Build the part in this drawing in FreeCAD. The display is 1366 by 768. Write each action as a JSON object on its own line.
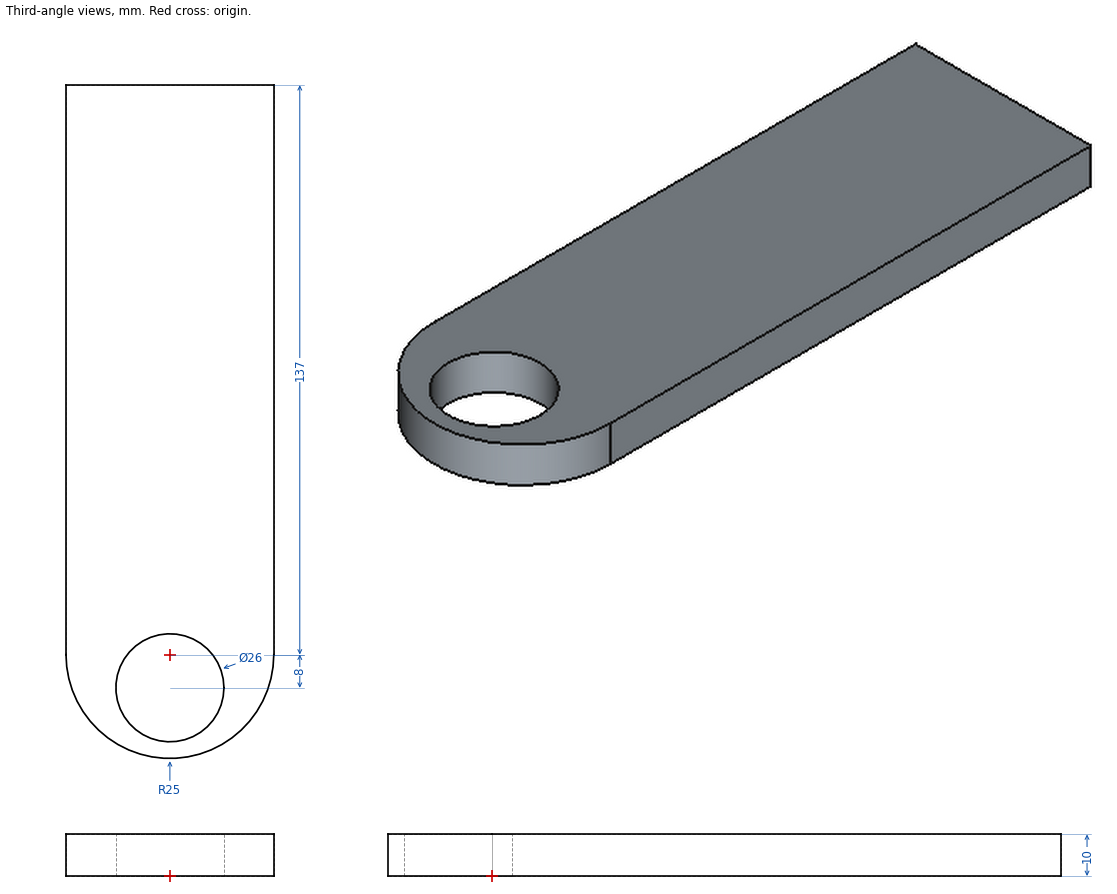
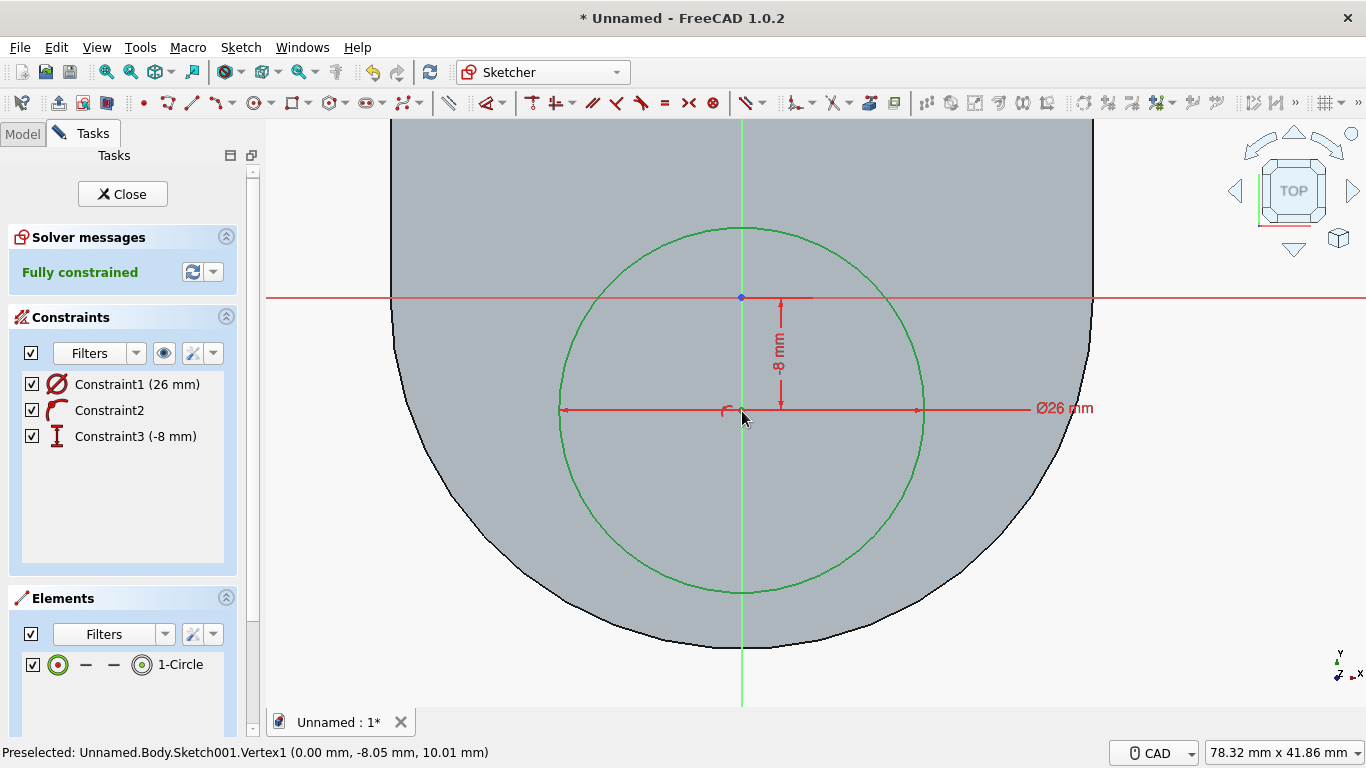
{"action": "left_click", "coordinate": [123, 194]}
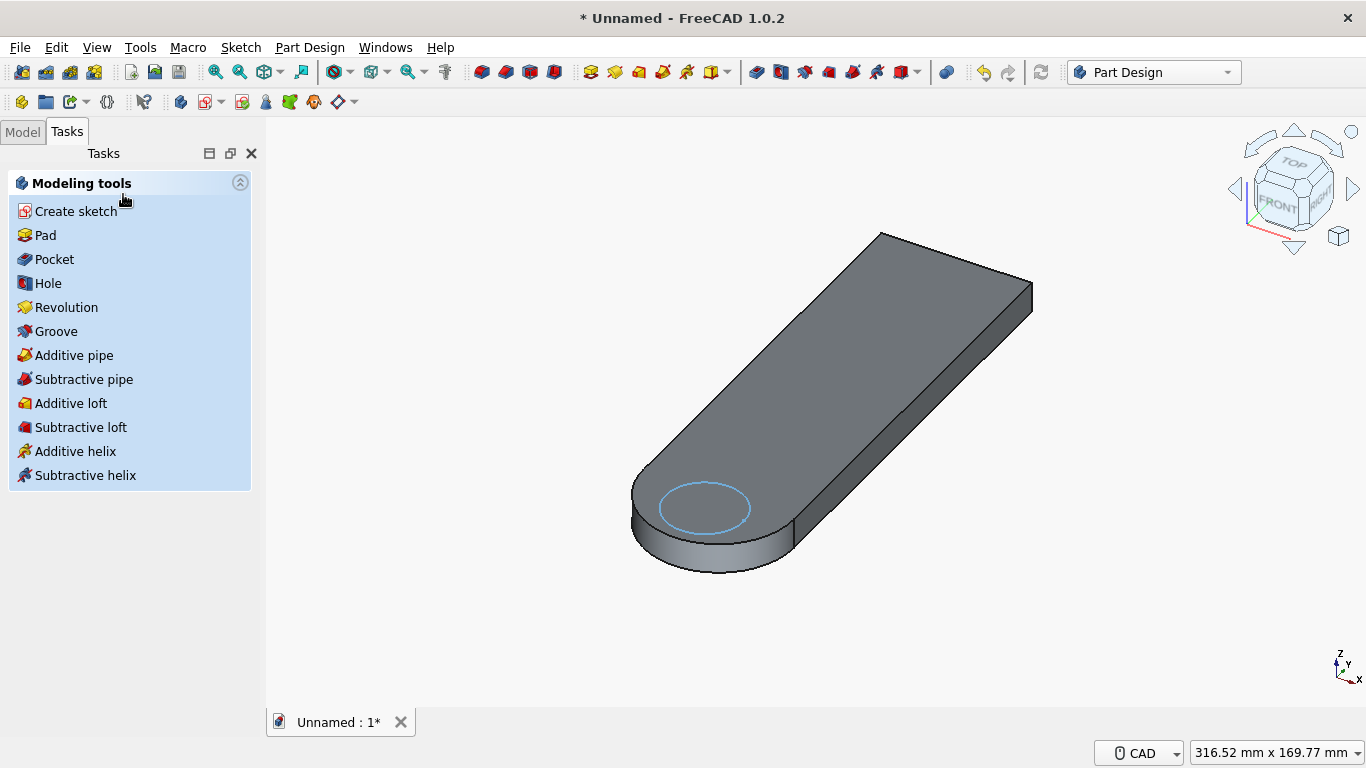
{"action": "left_click", "coordinate": [758, 72]}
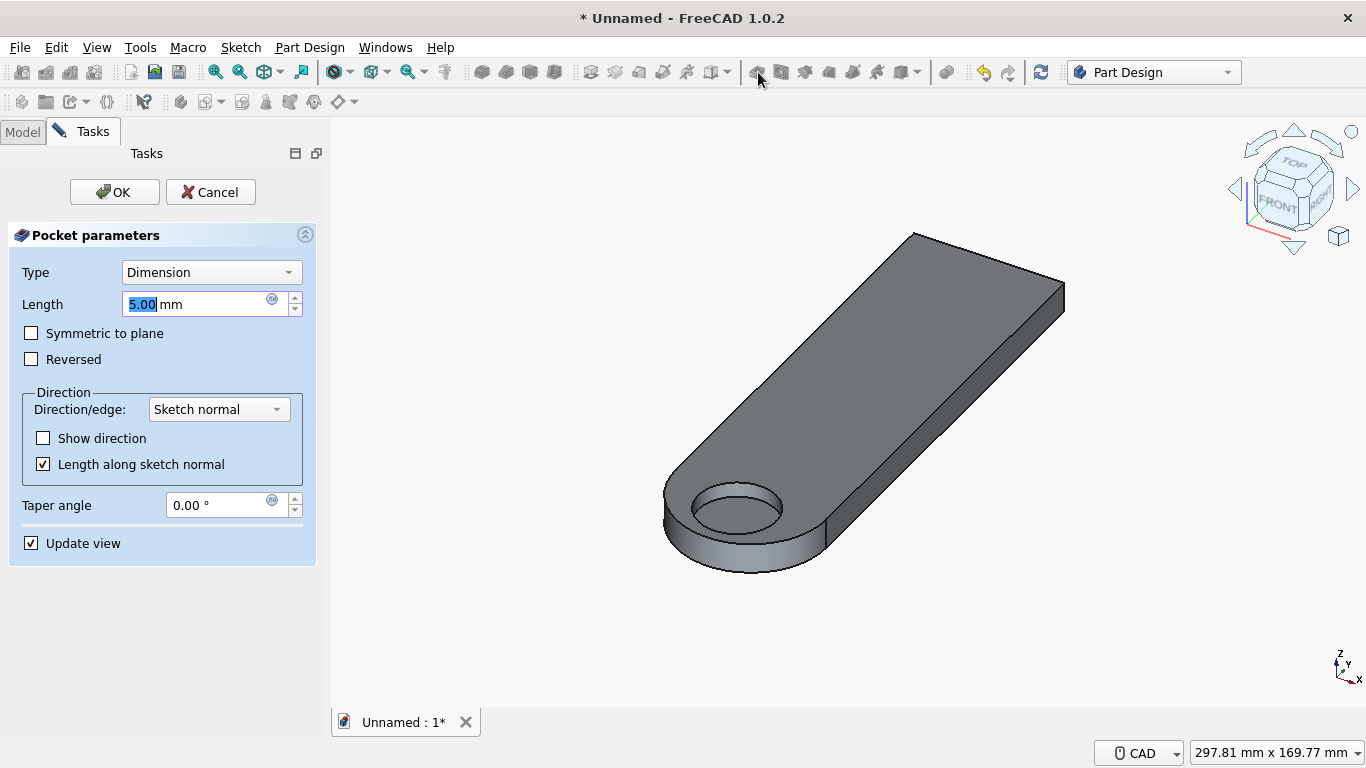
{"action": "left_click", "coordinate": [212, 272]}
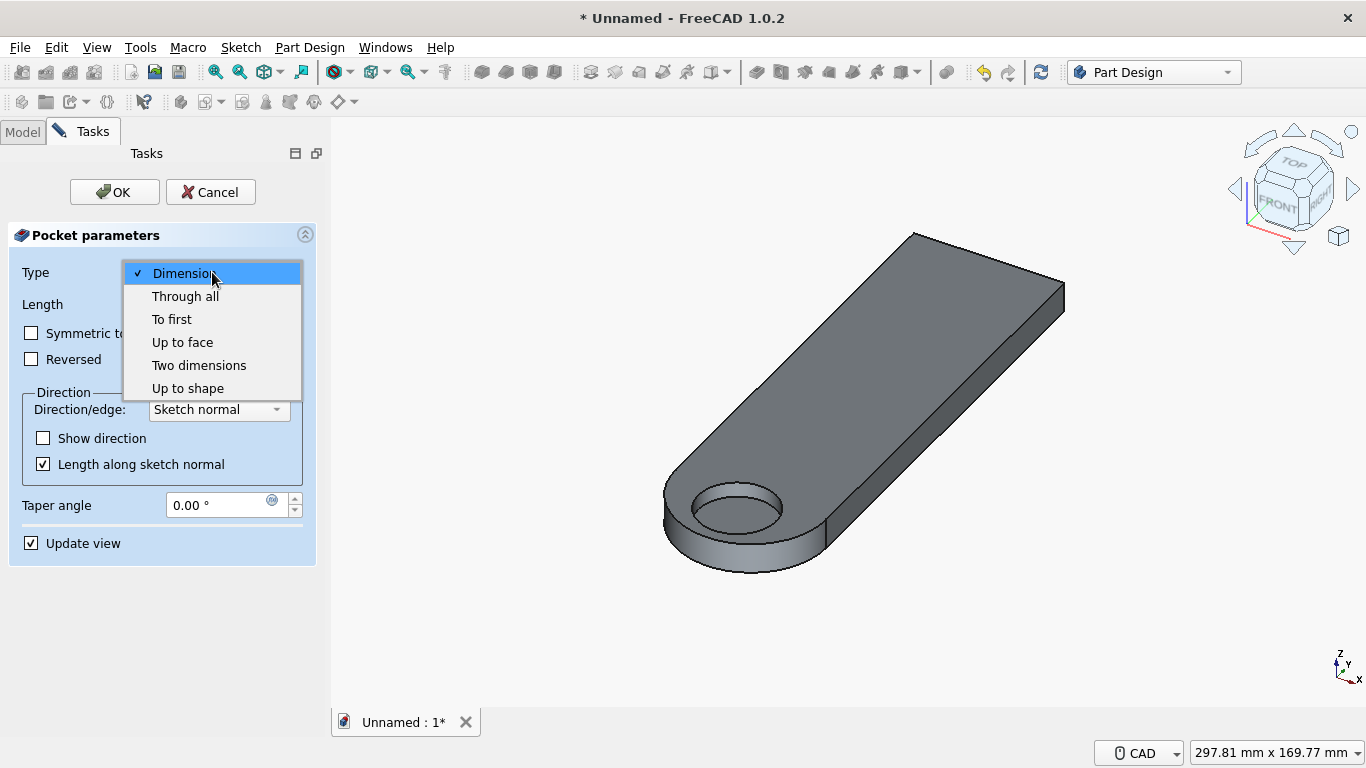
{"action": "left_click", "coordinate": [212, 296]}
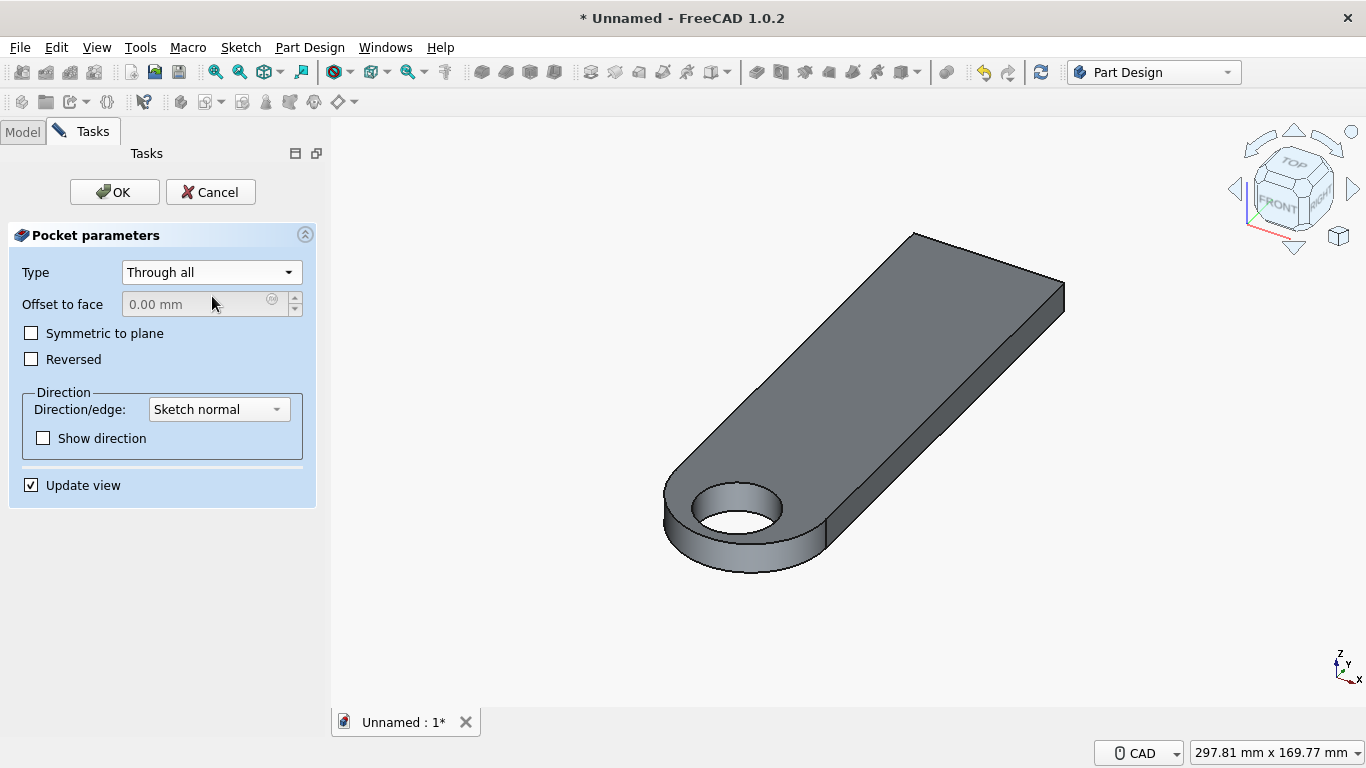
{"action": "left_click", "coordinate": [115, 192]}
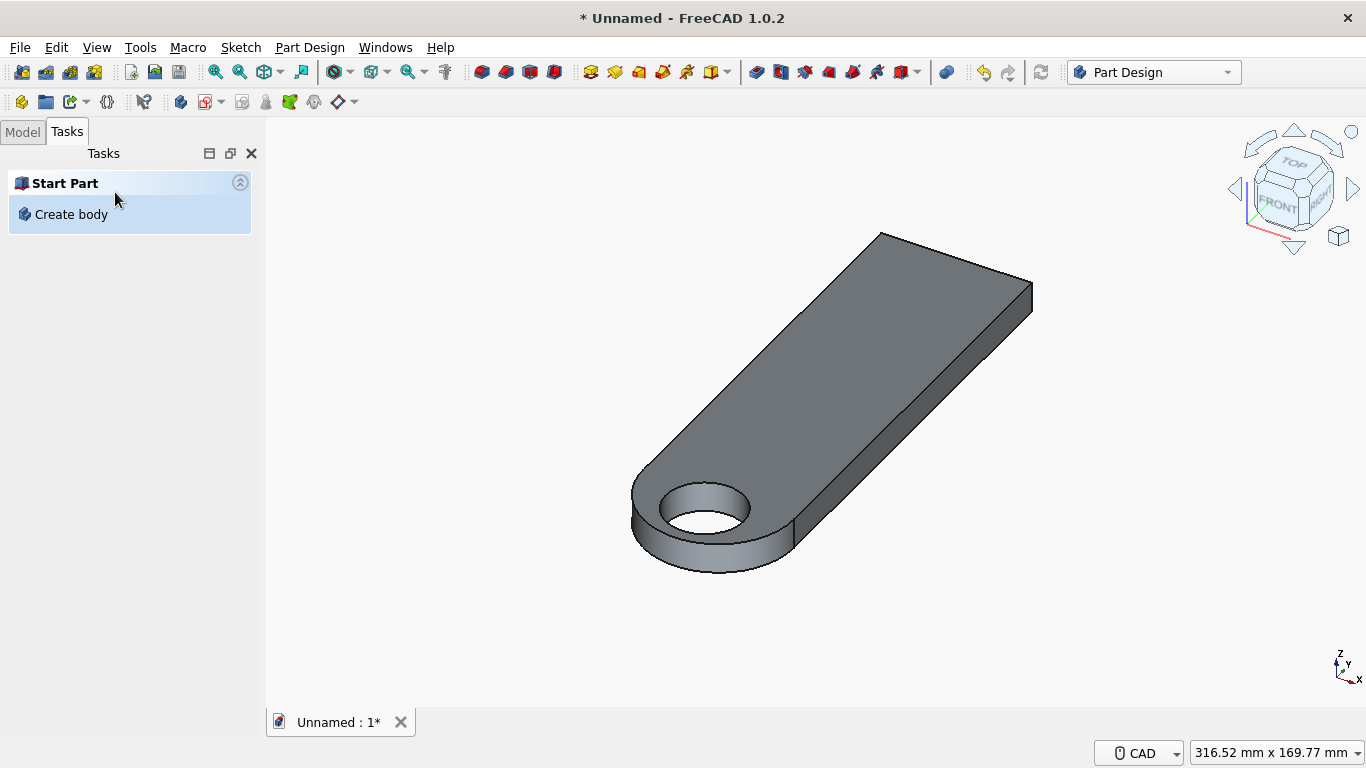
{"action": "key", "text": "0"}